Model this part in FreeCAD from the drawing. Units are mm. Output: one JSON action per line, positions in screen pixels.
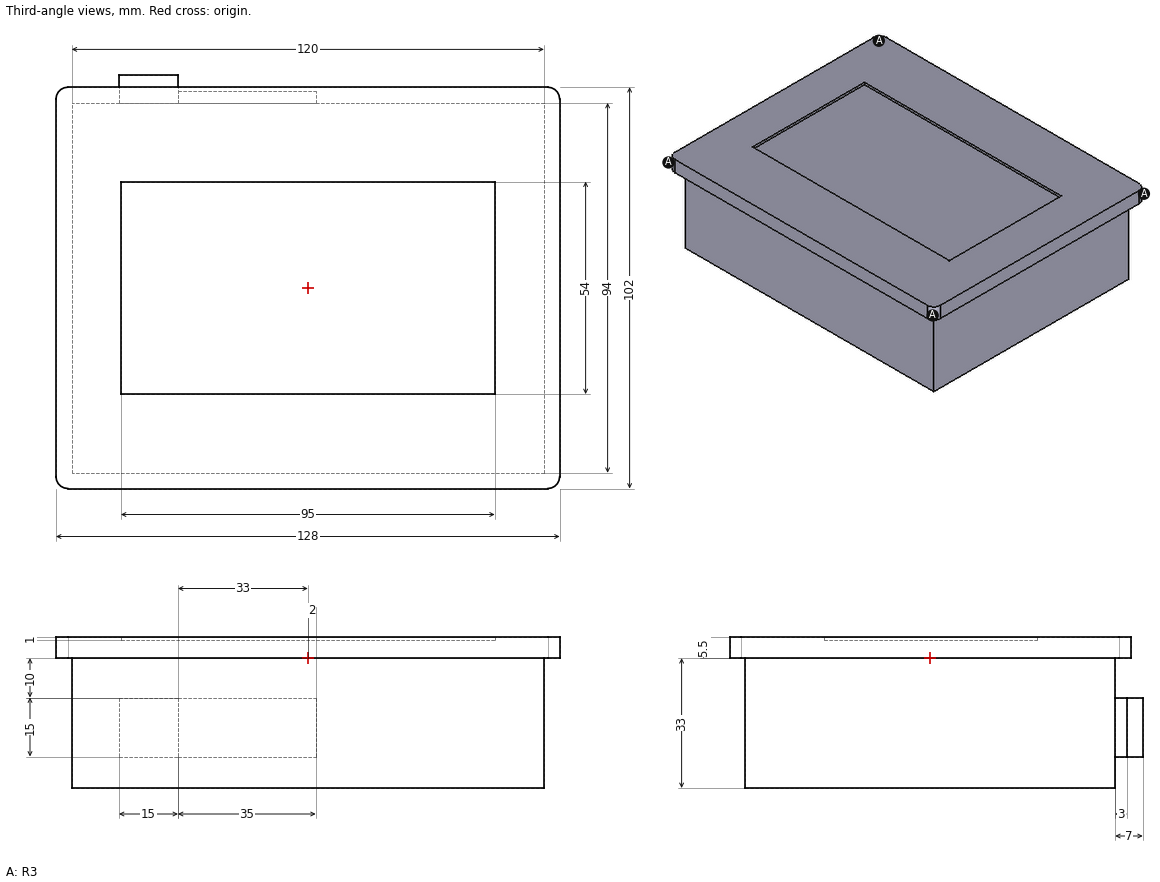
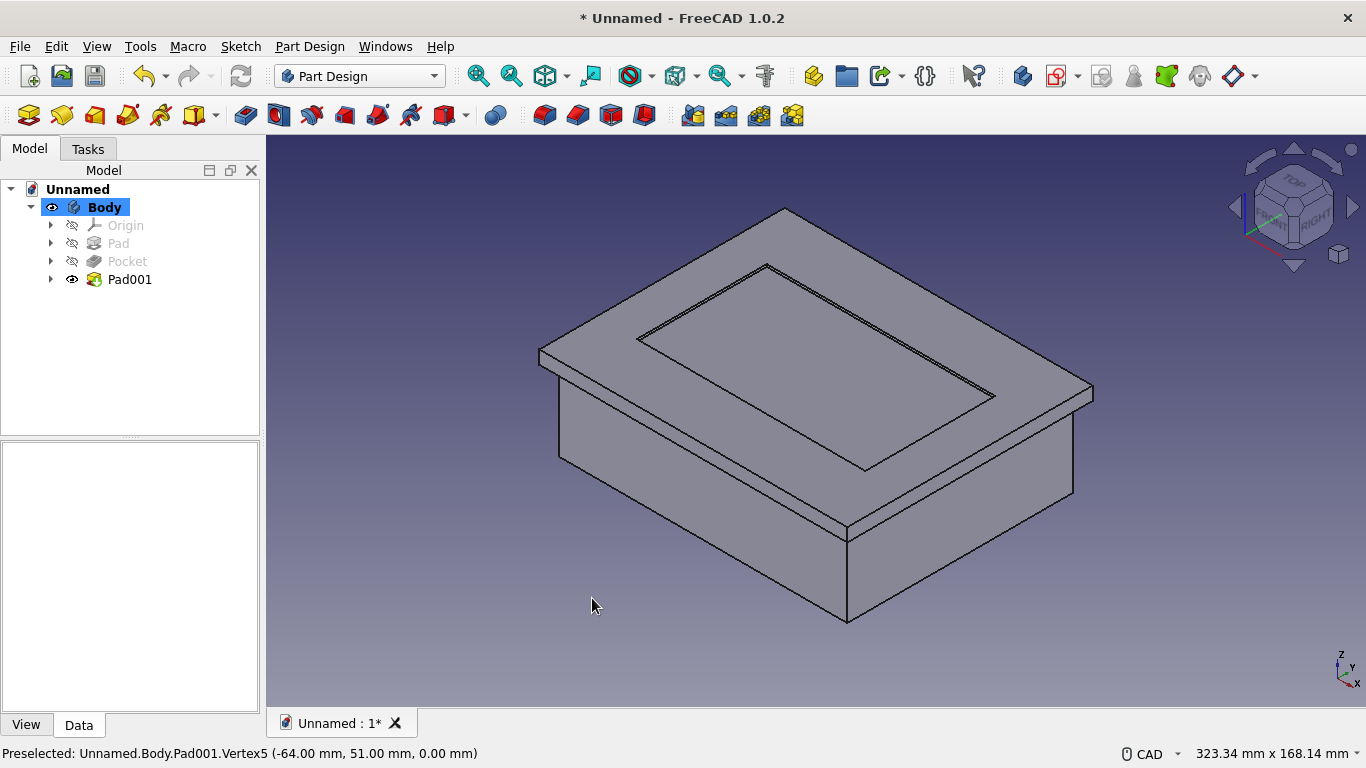
{"action": "left_click", "coordinate": [847, 534]}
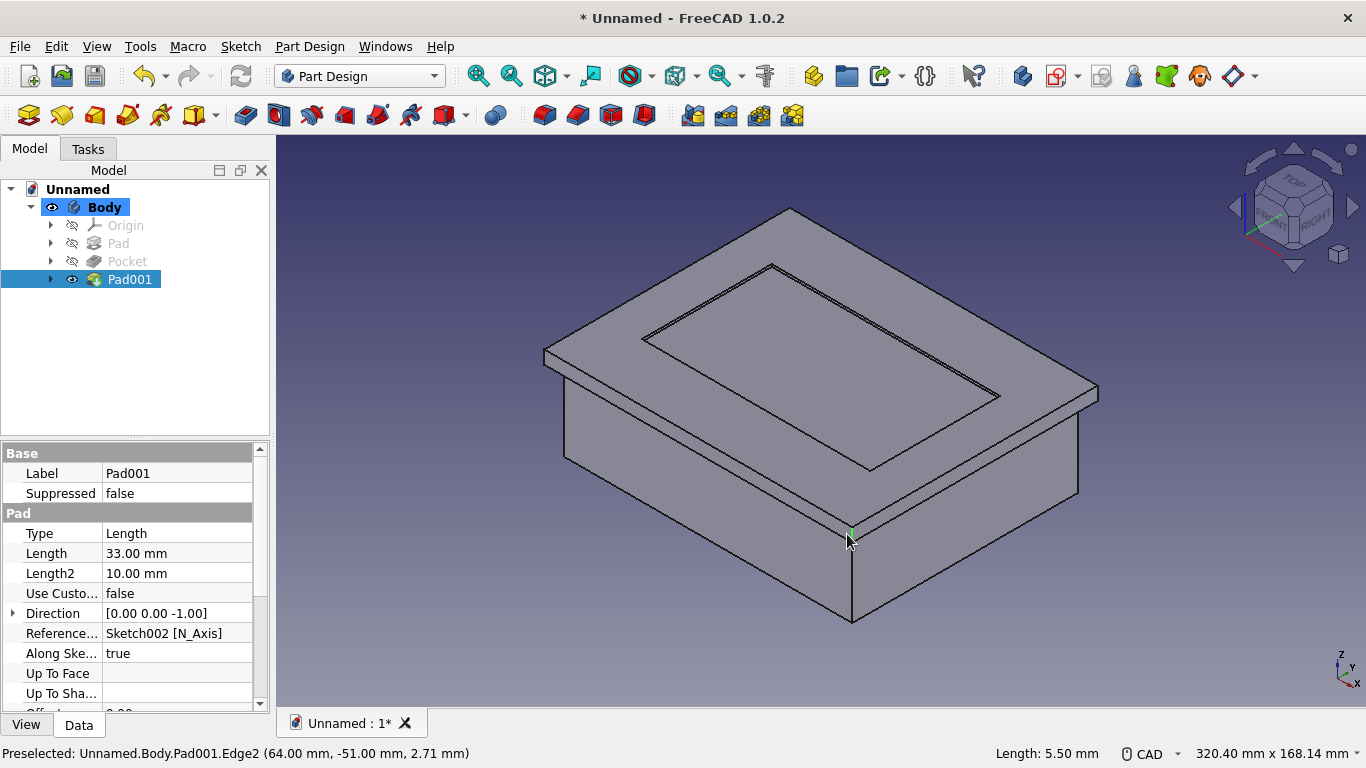
{"action": "scroll", "coordinate": [790, 214], "scroll_direction": "up", "scroll_amount": 4}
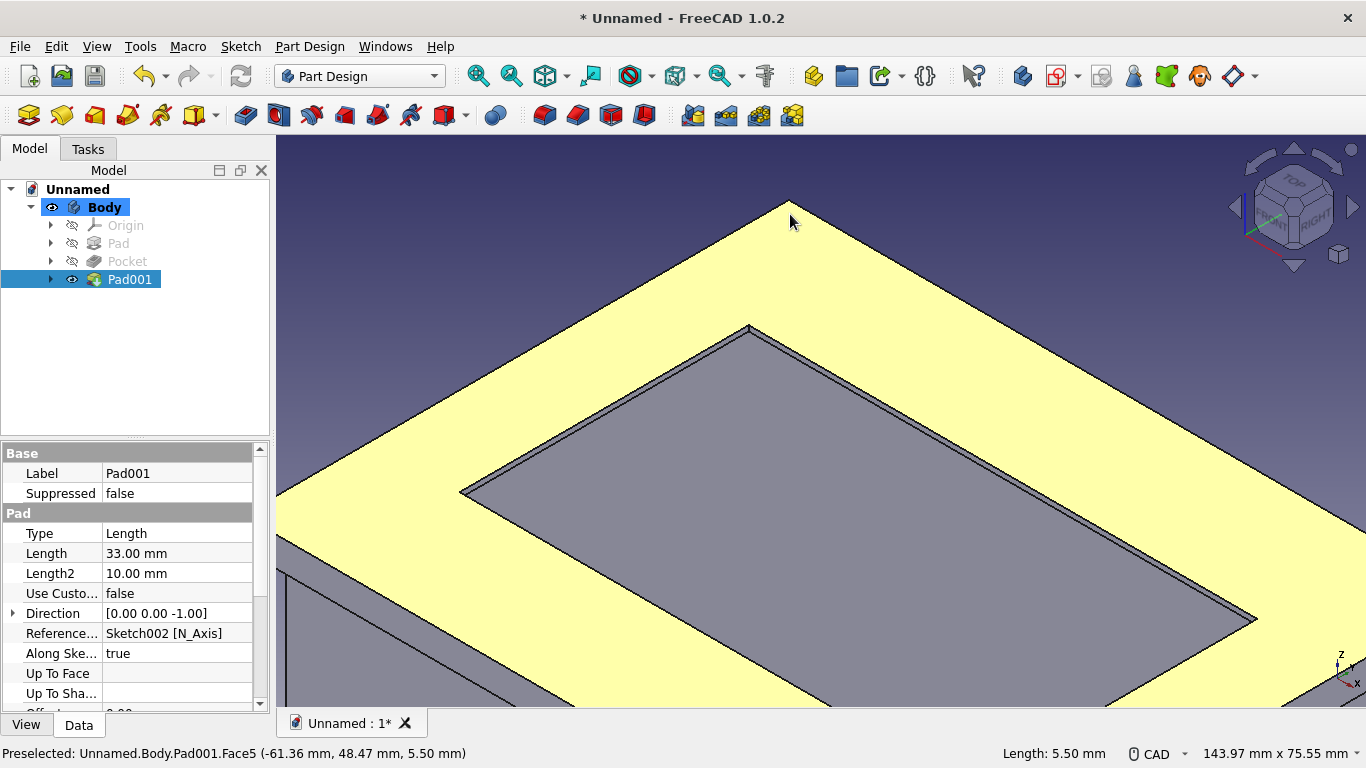
{"action": "key", "text": "v f"}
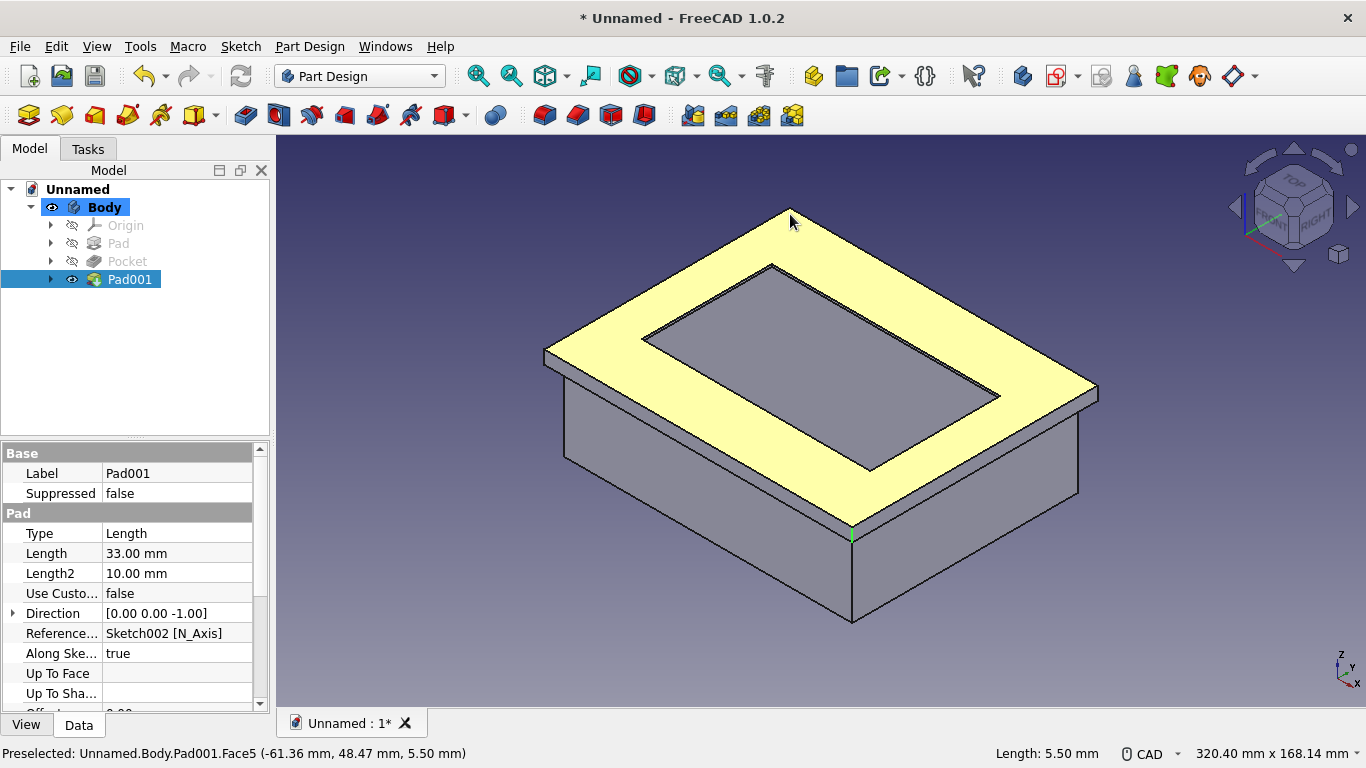
{"action": "key", "text": "2"}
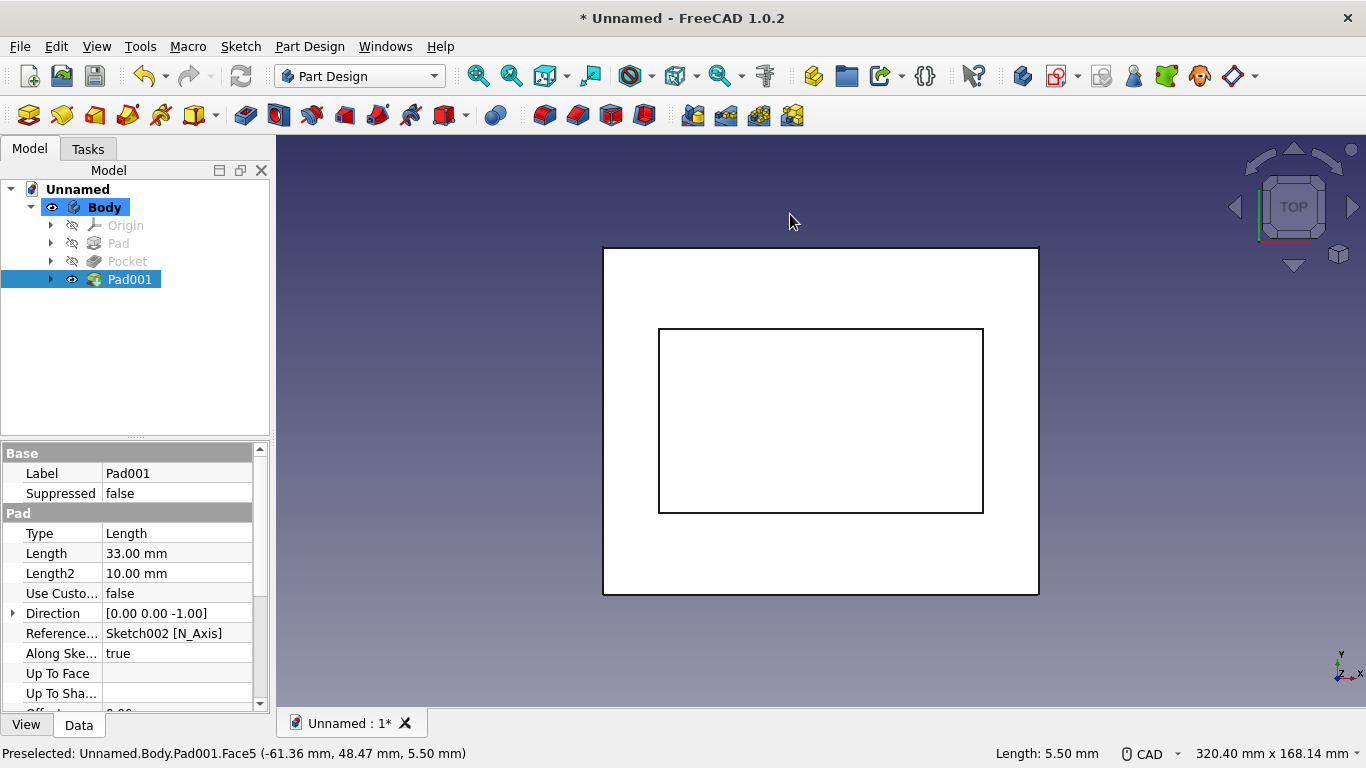
{"action": "scroll", "coordinate": [603, 246], "scroll_direction": "up", "scroll_amount": 4}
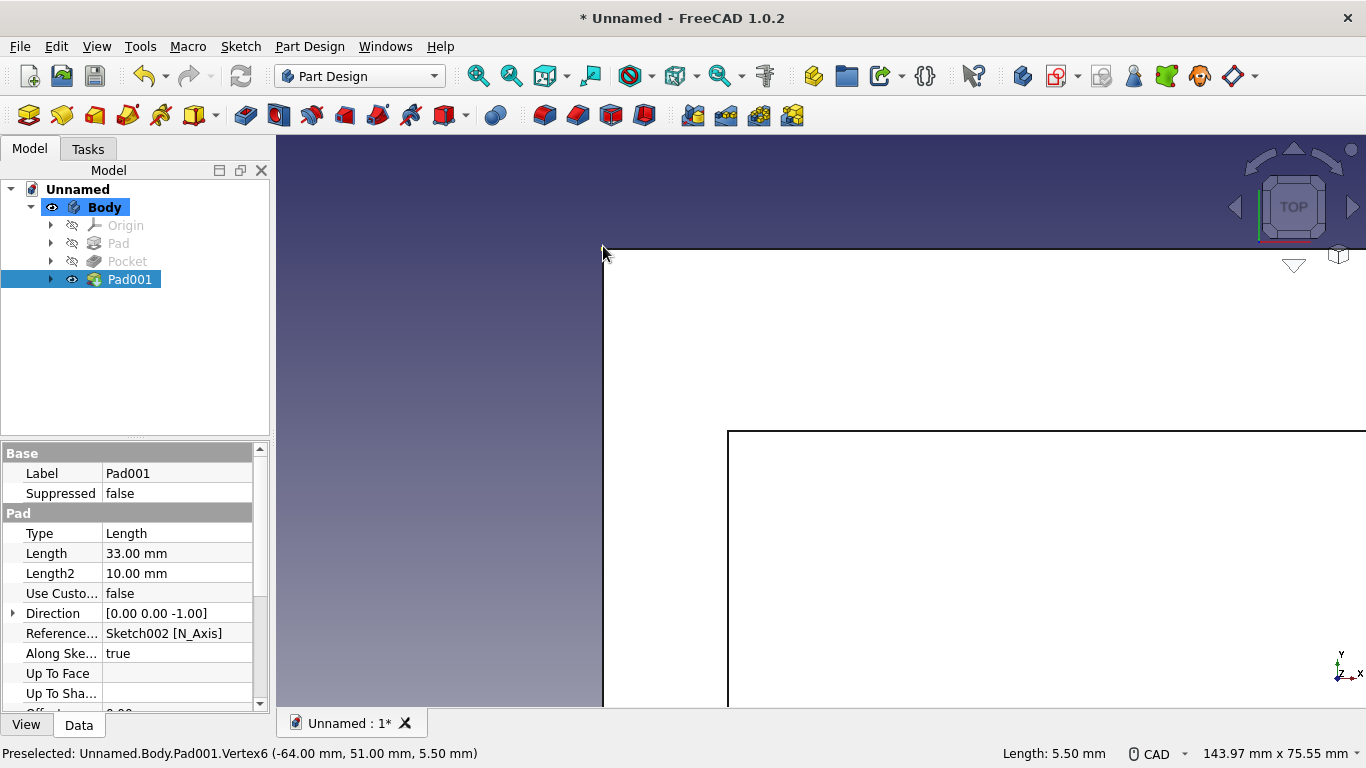
{"action": "left_click", "coordinate": [479, 76]}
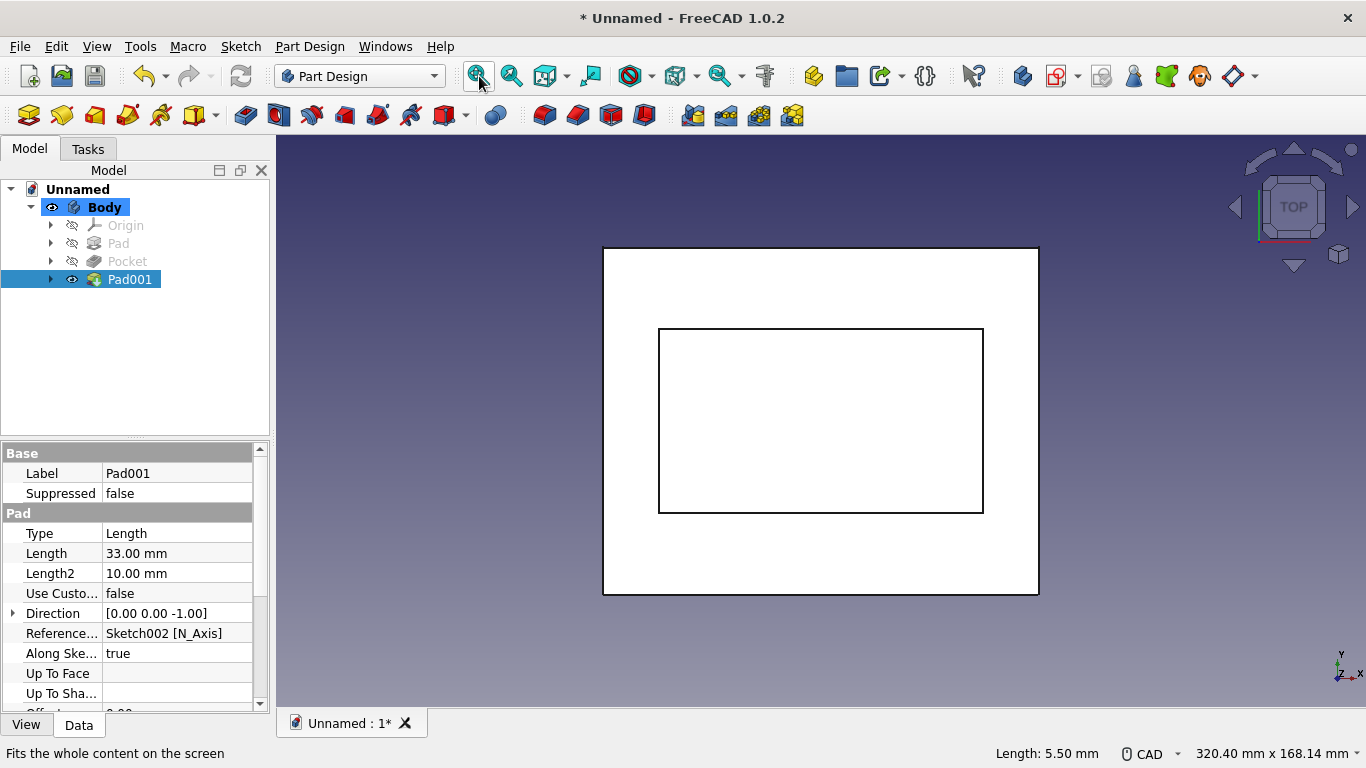
{"action": "key", "text": "1"}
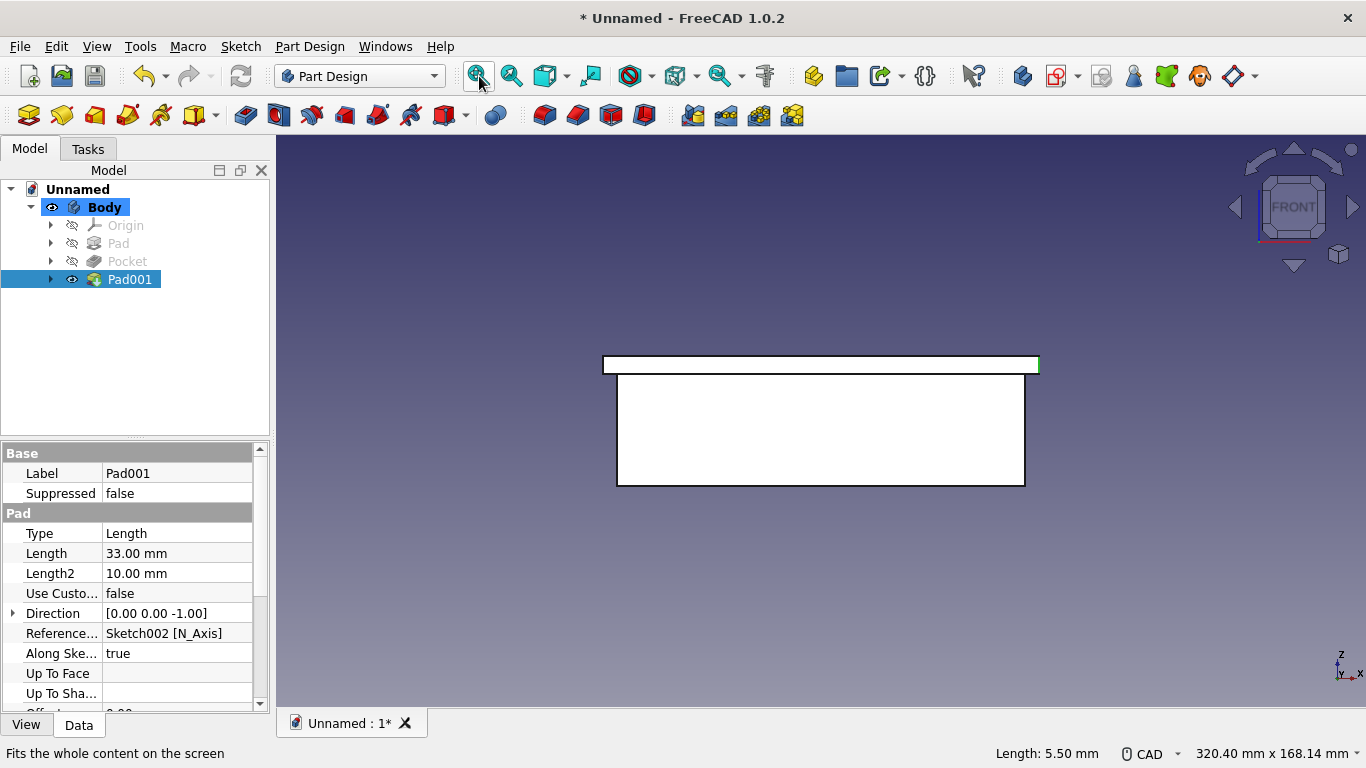
{"action": "key", "text": "v f"}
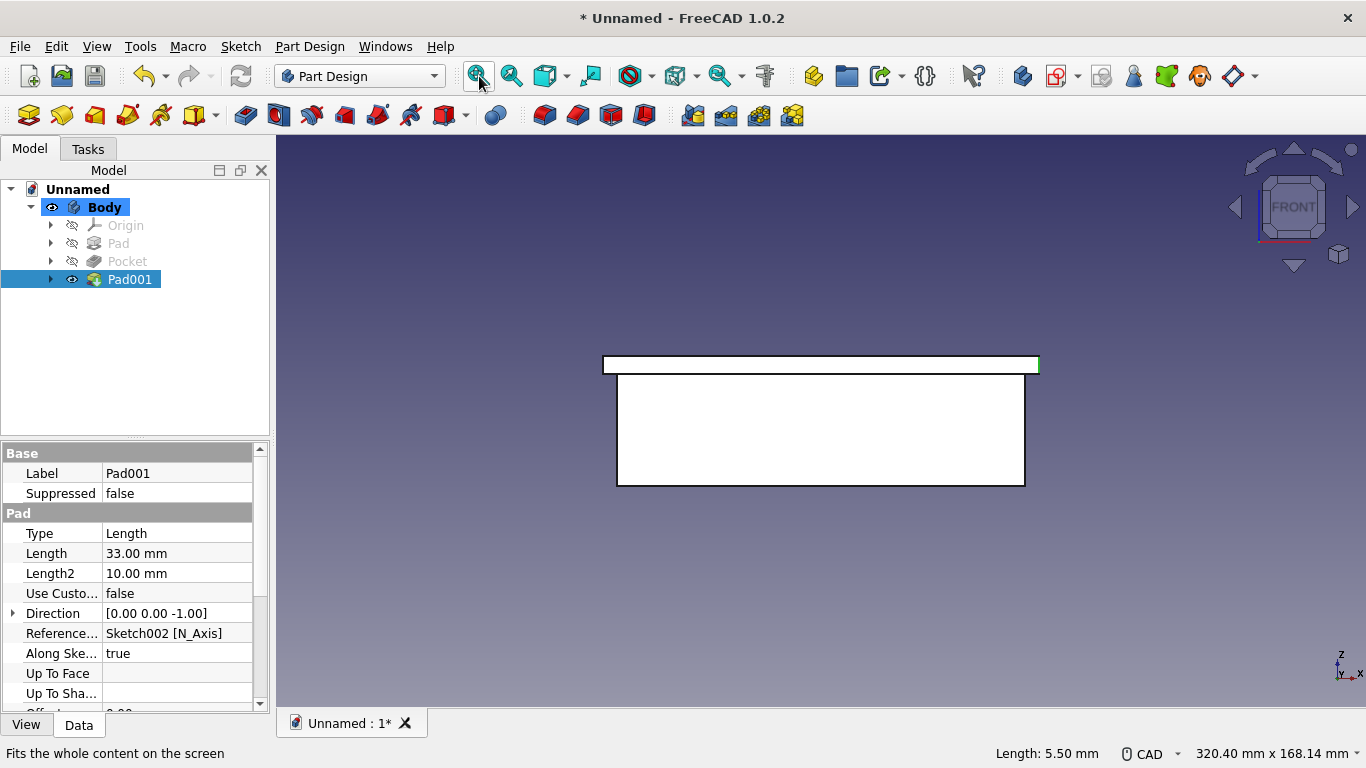
{"action": "left_click", "coordinate": [603, 364], "text": "ctrl"}